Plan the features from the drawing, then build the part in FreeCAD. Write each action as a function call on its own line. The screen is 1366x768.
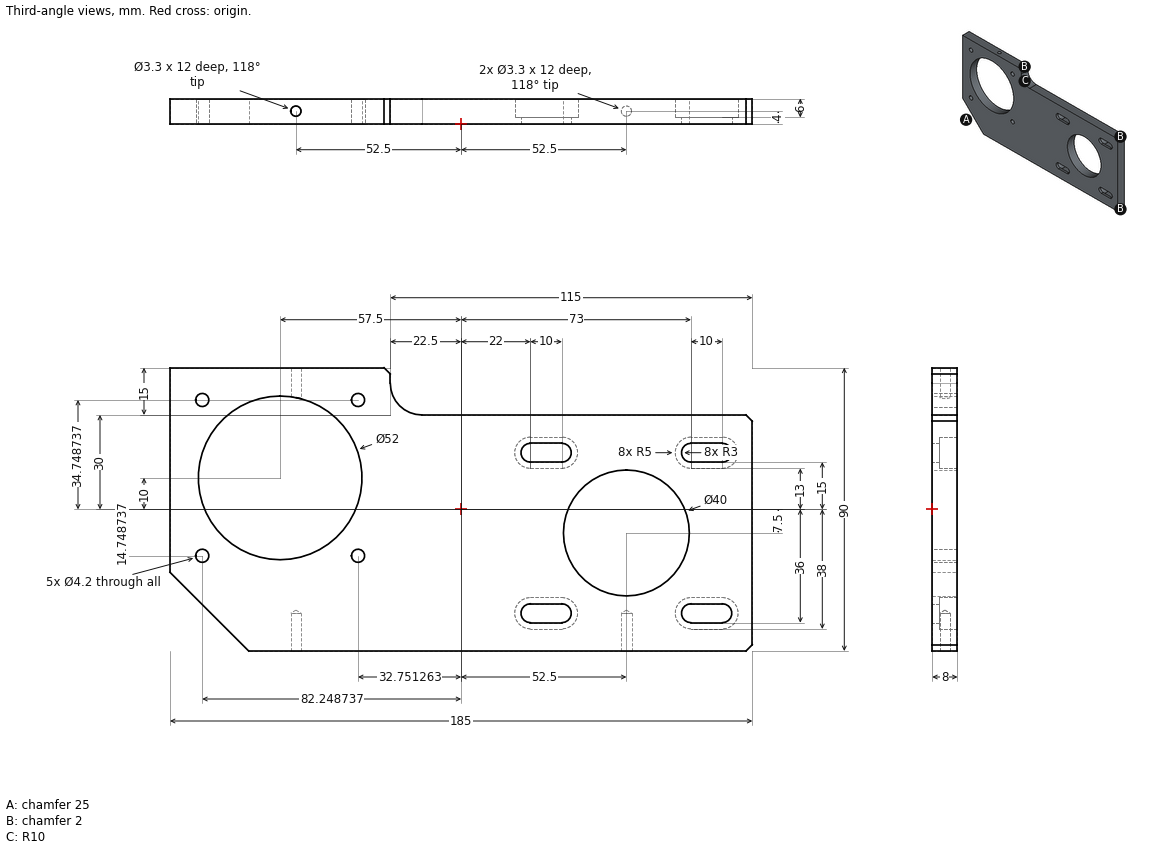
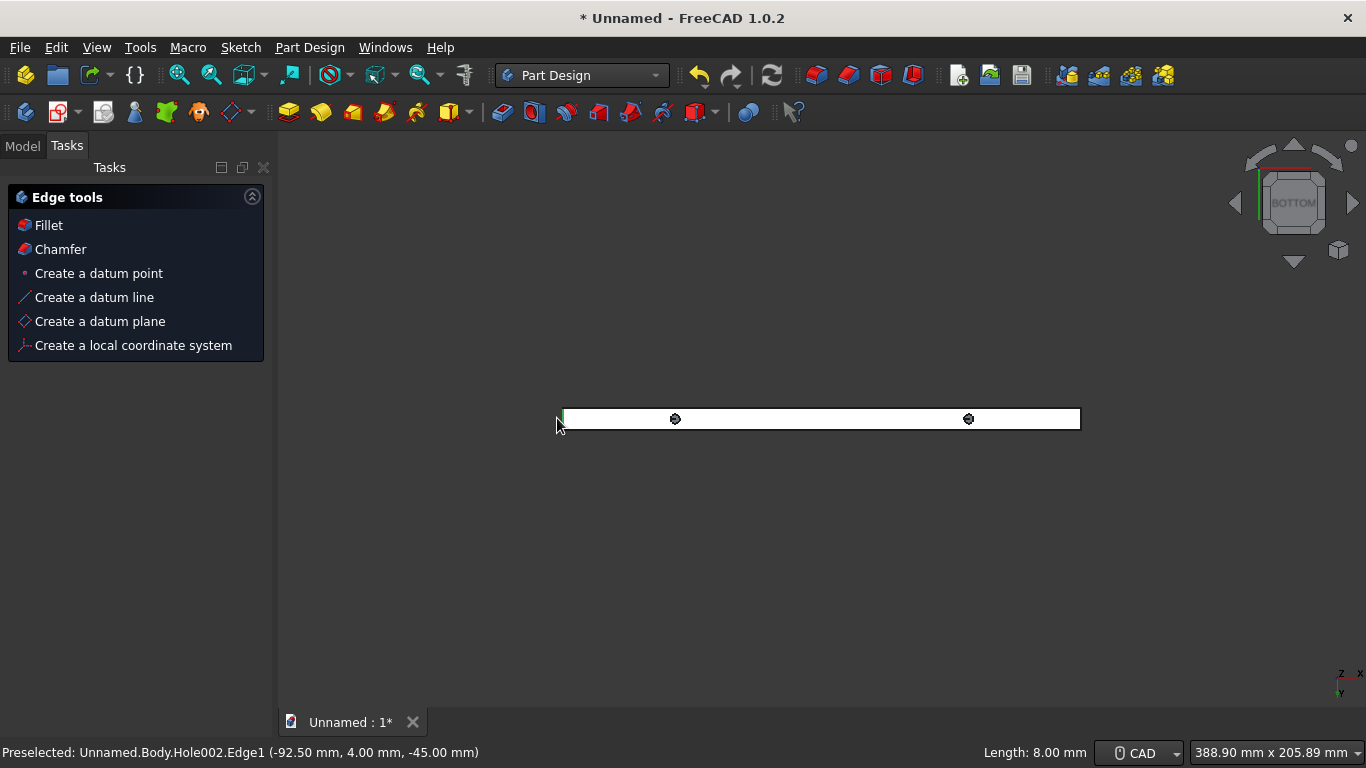
click(850, 76)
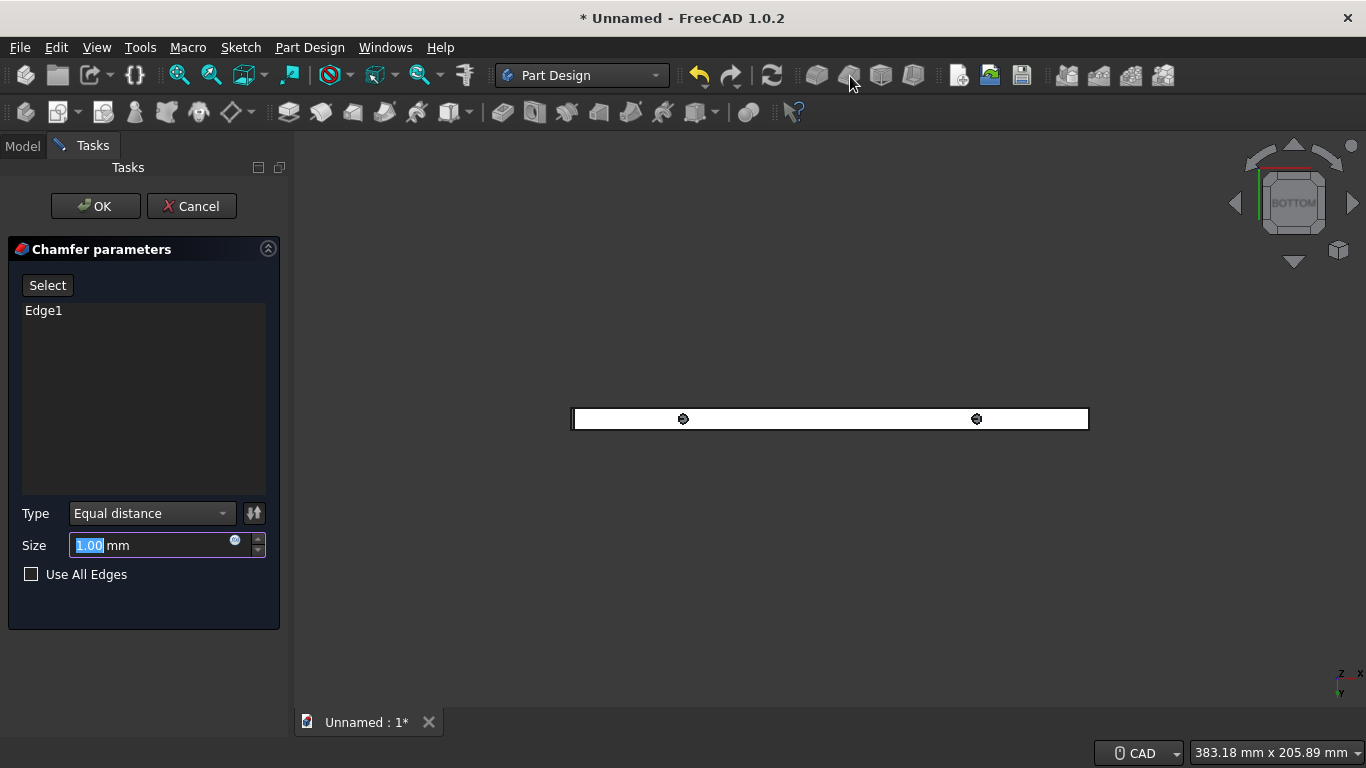
text(25)
key(Tab)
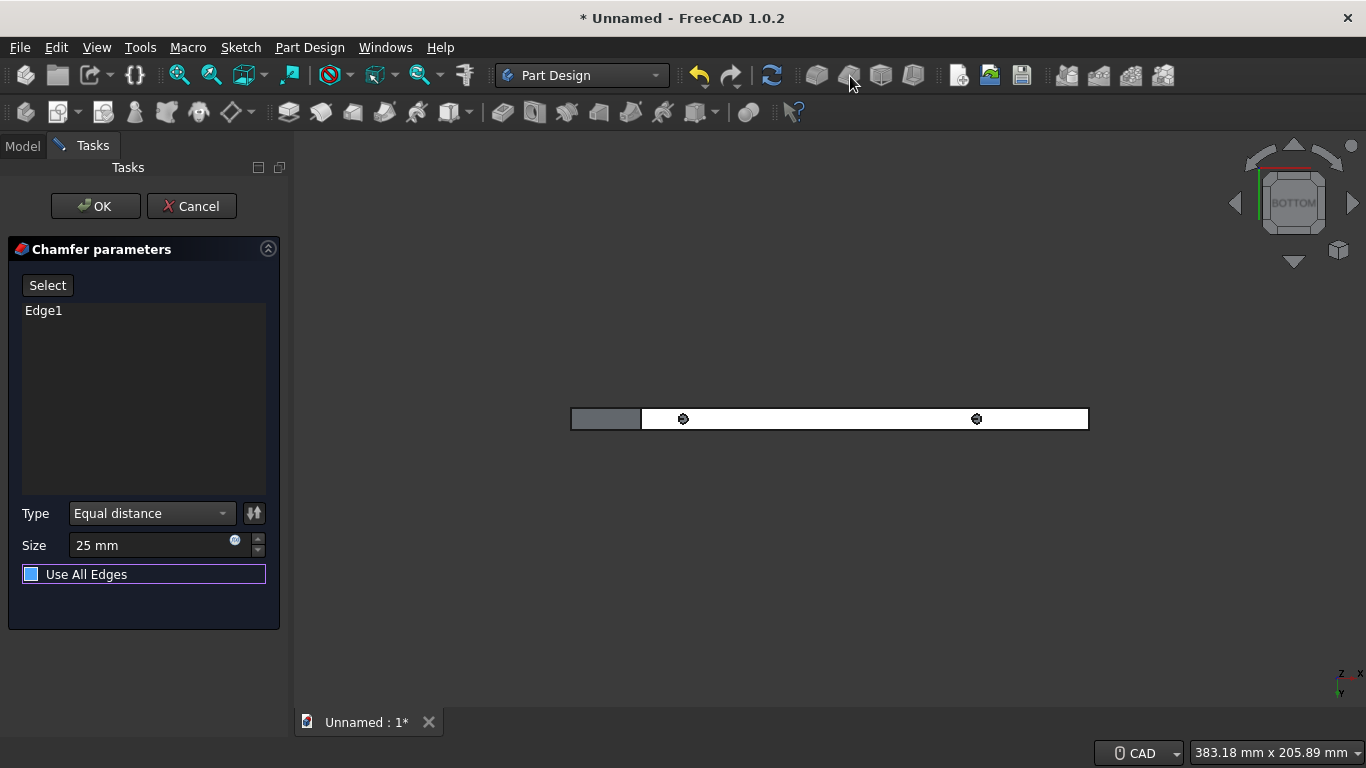
click(96, 206)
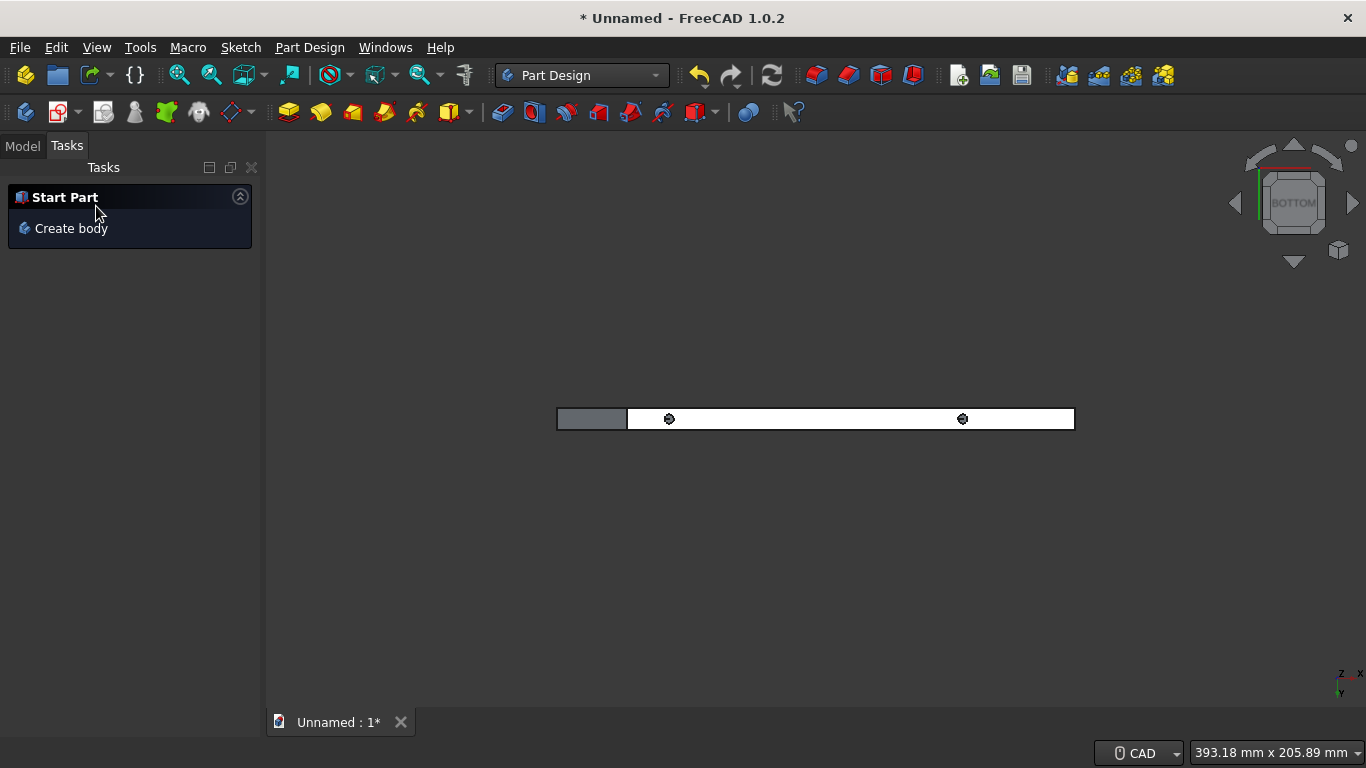
click(1075, 418)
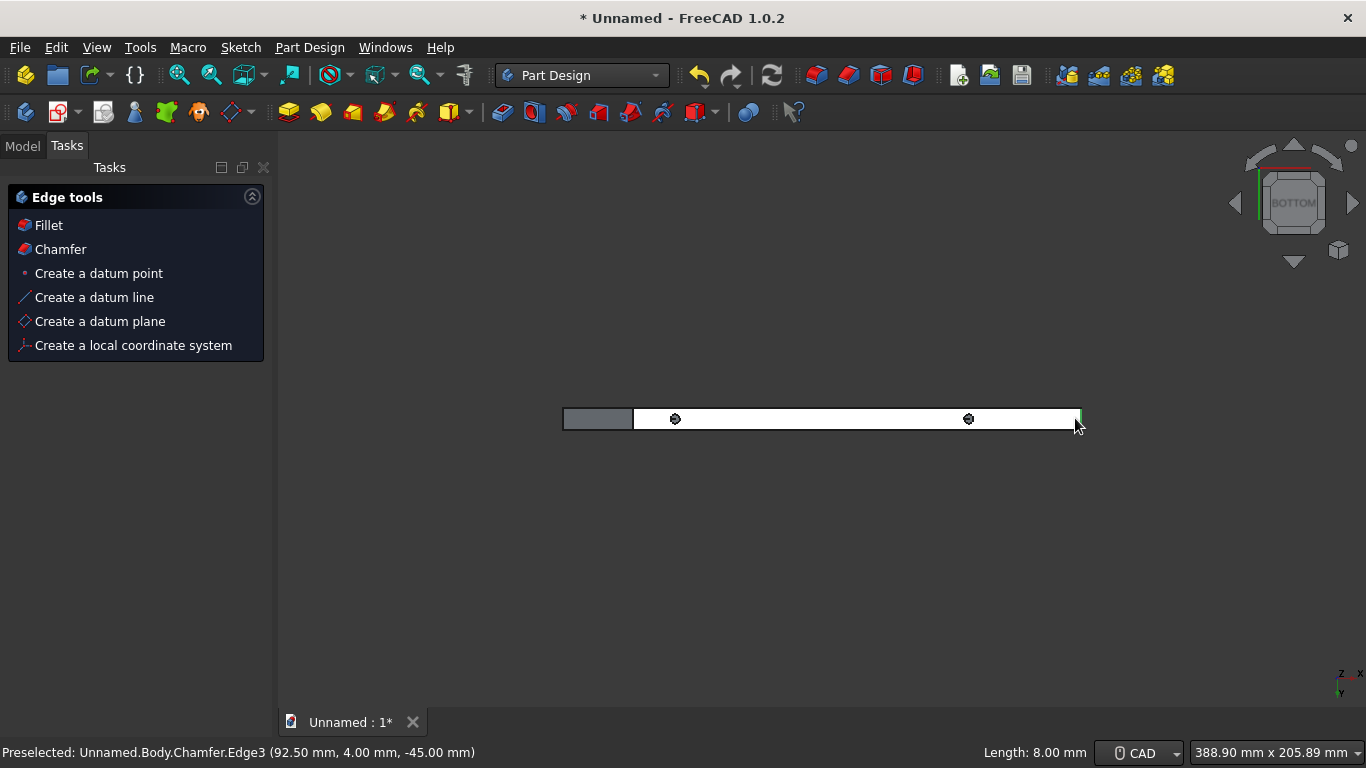
key(0)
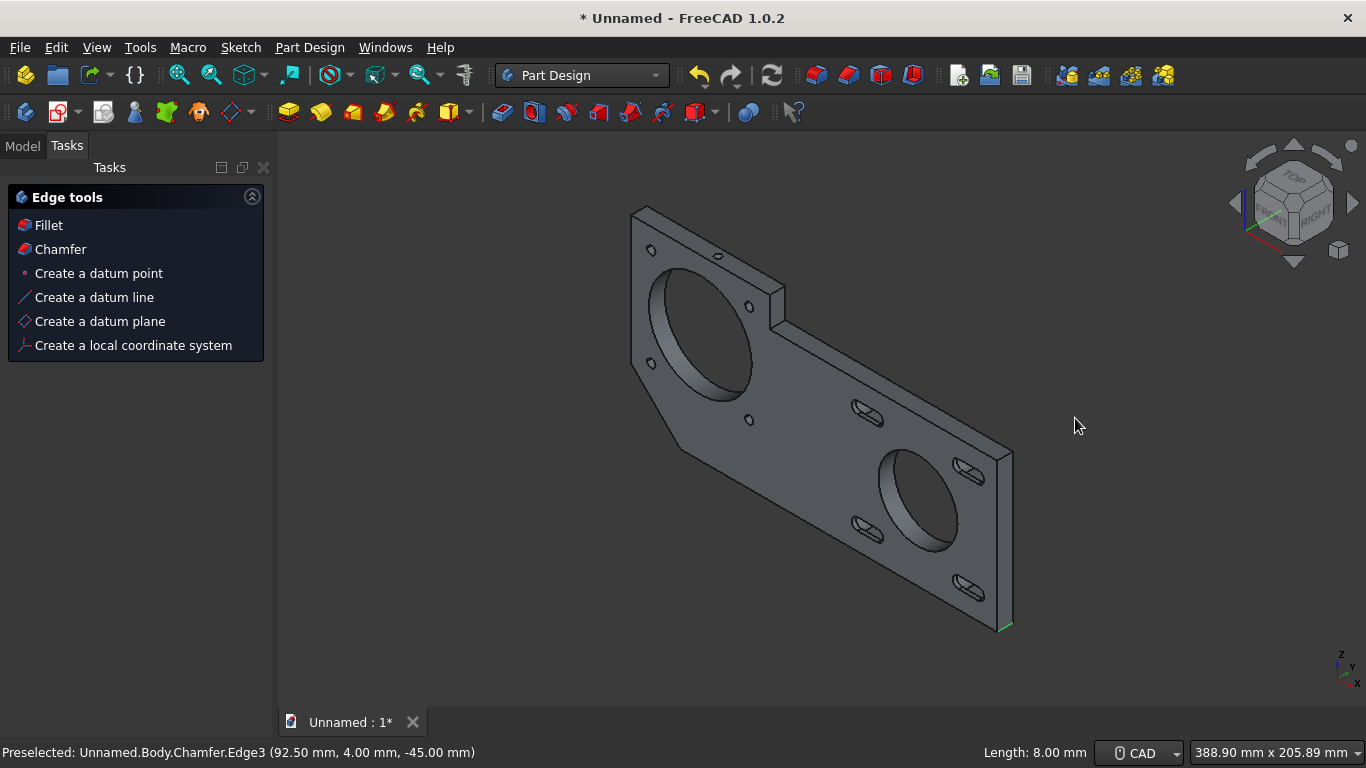
click(1005, 455, ctrl)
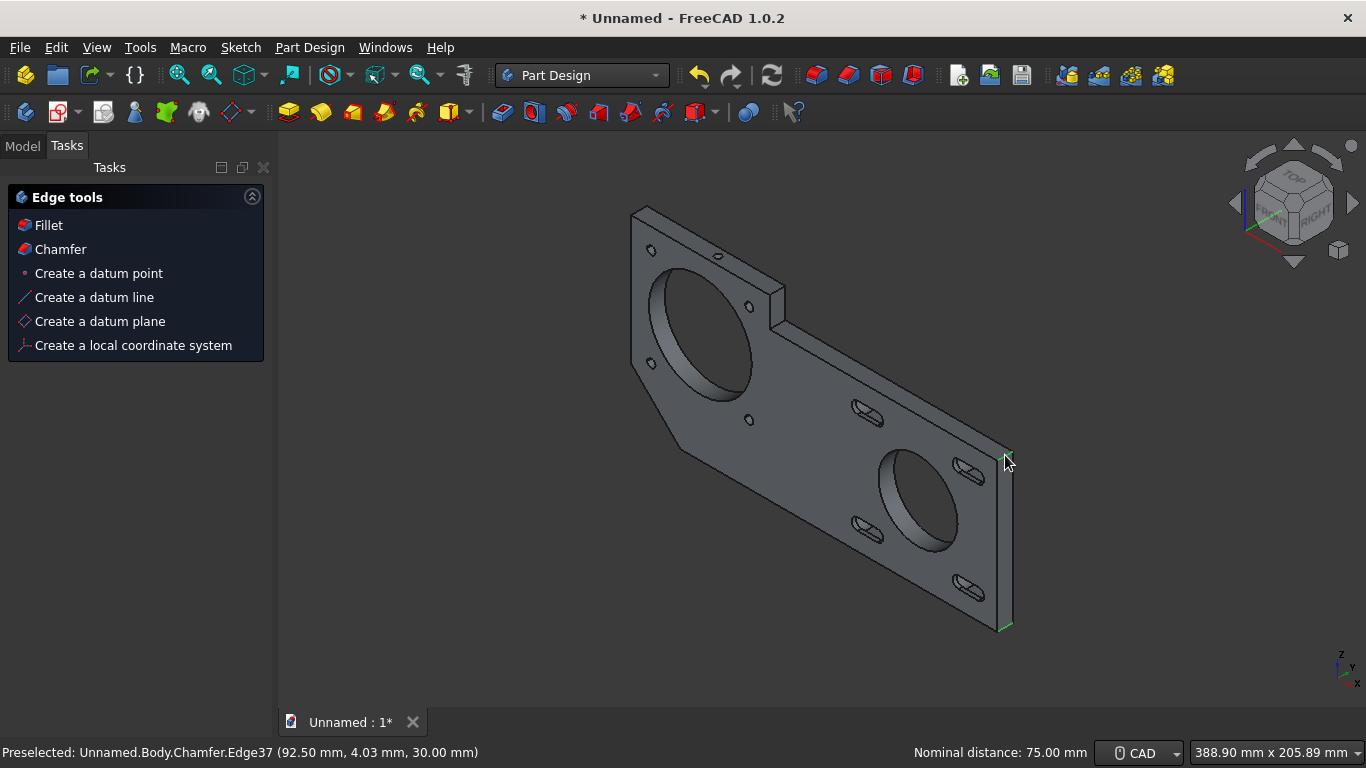
click(777, 290, ctrl)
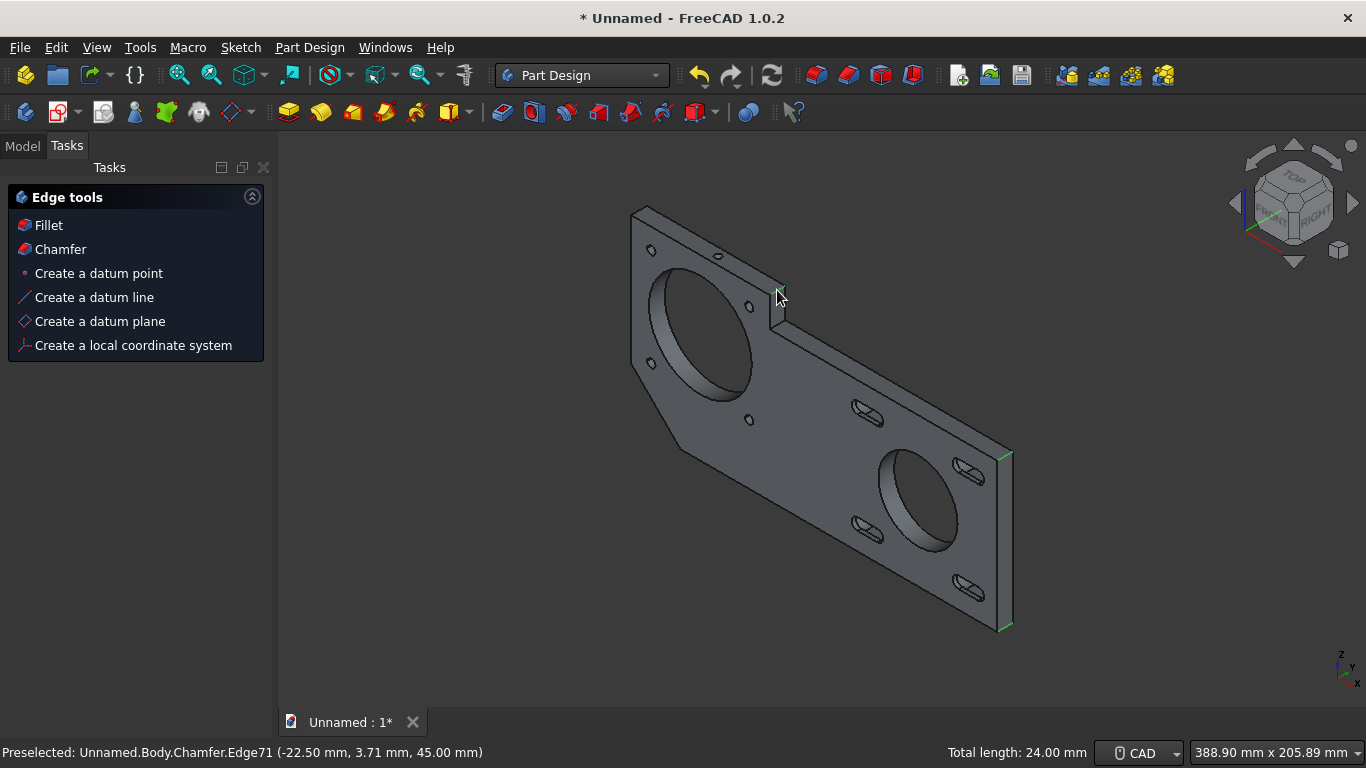
click(850, 76)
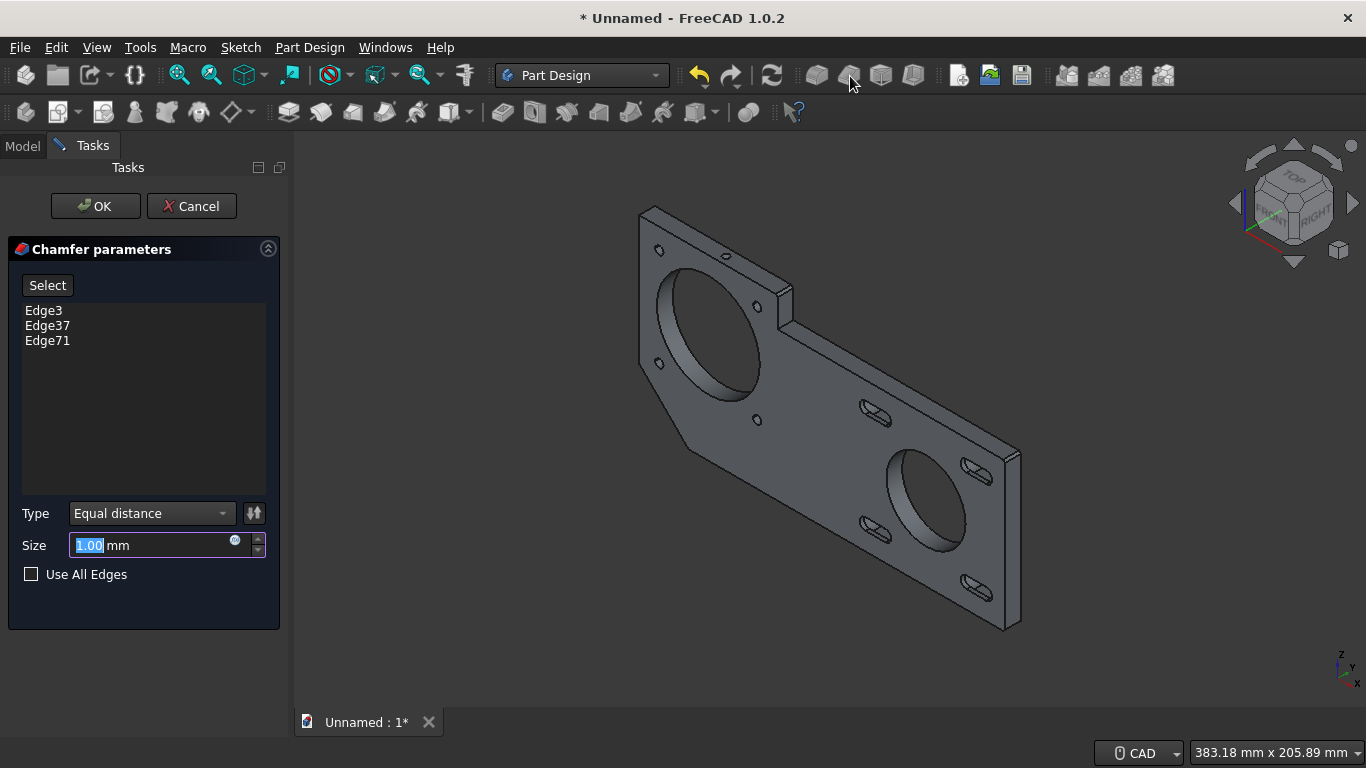
text(2)
key(Tab)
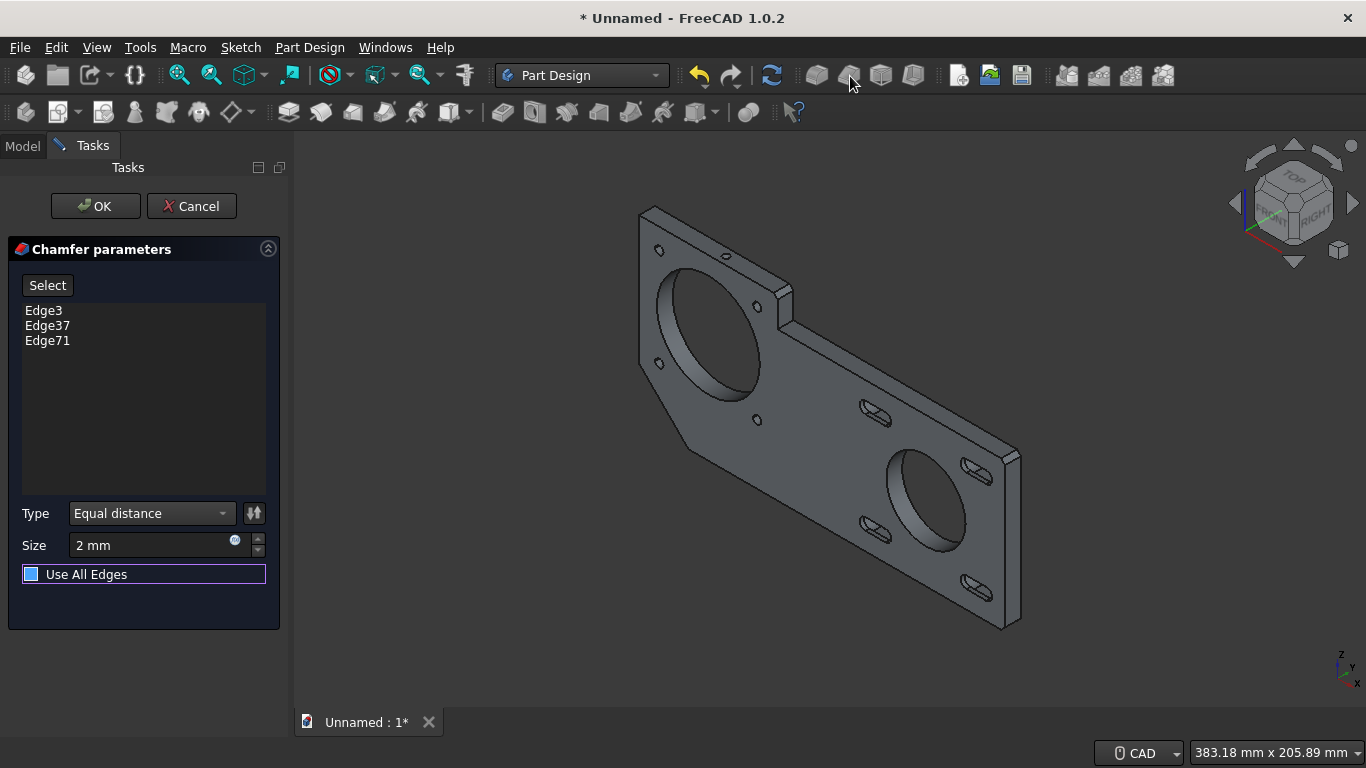
click(96, 206)